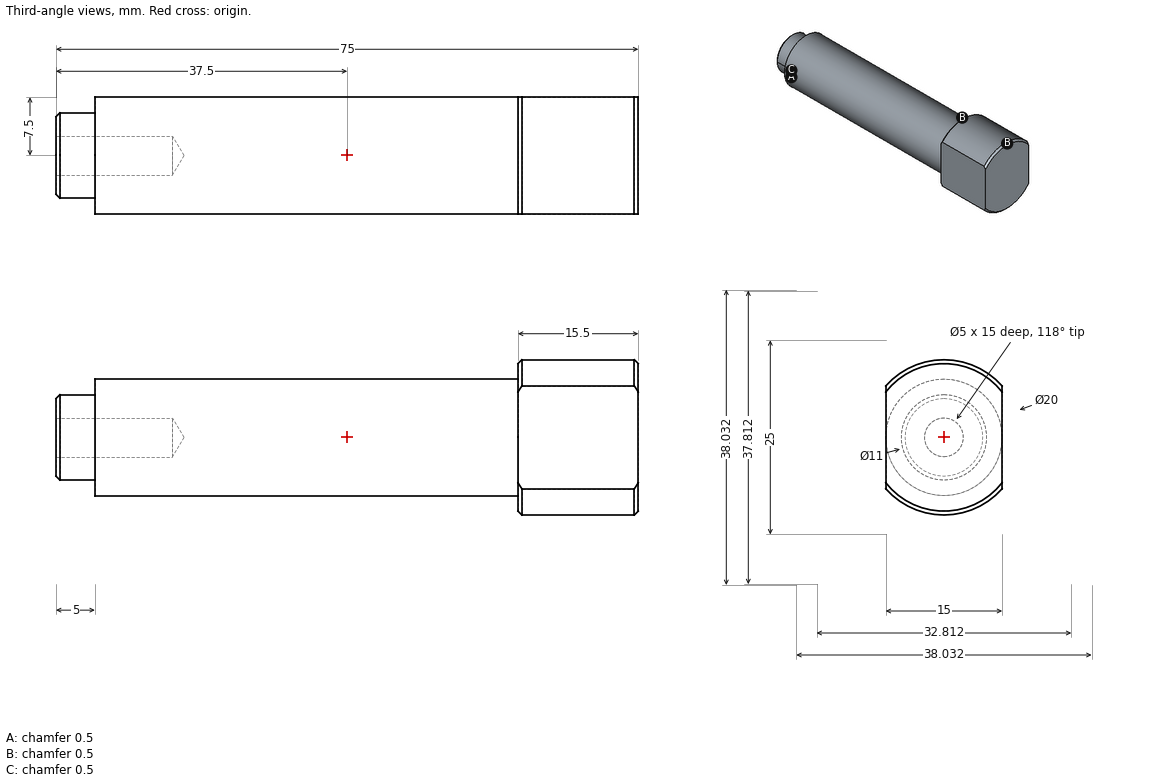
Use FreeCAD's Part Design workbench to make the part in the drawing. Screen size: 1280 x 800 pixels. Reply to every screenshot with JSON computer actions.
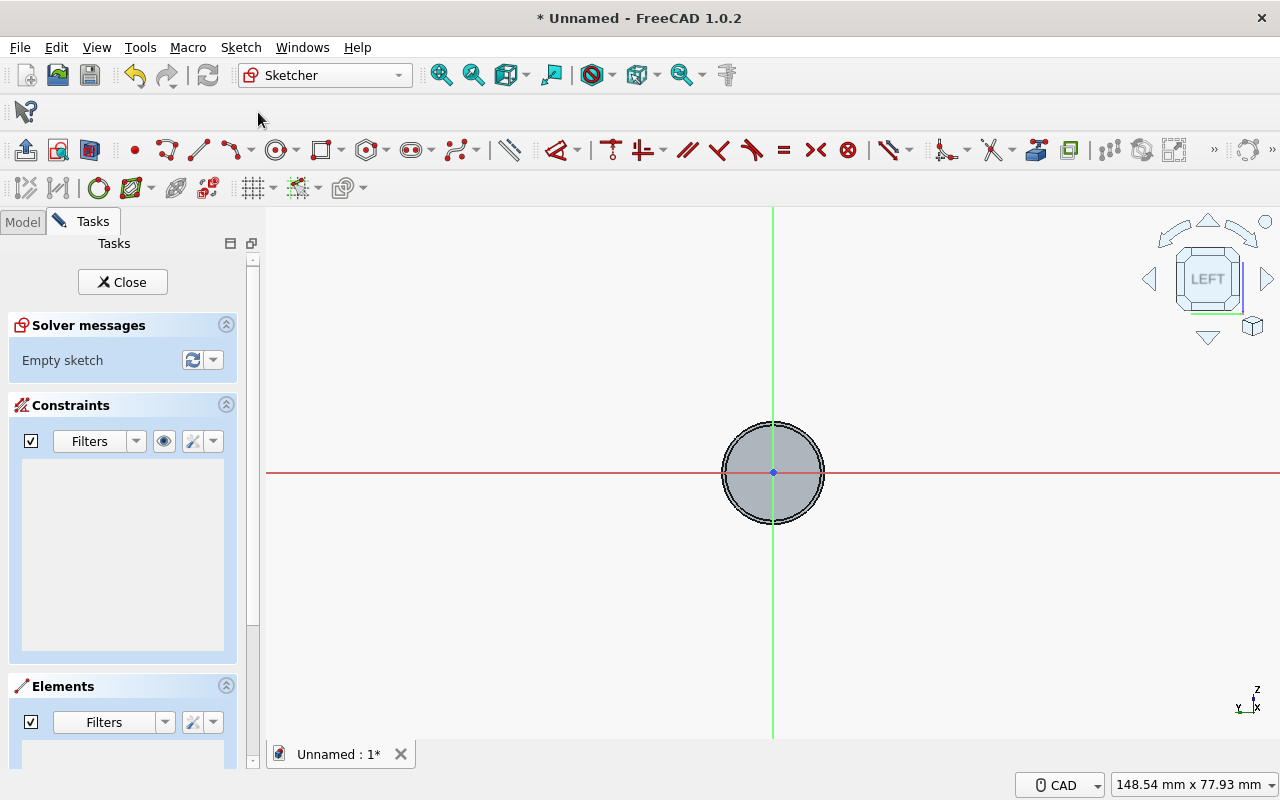
{"action": "scroll", "coordinate": [782, 473], "scroll_direction": "up", "scroll_amount": 11}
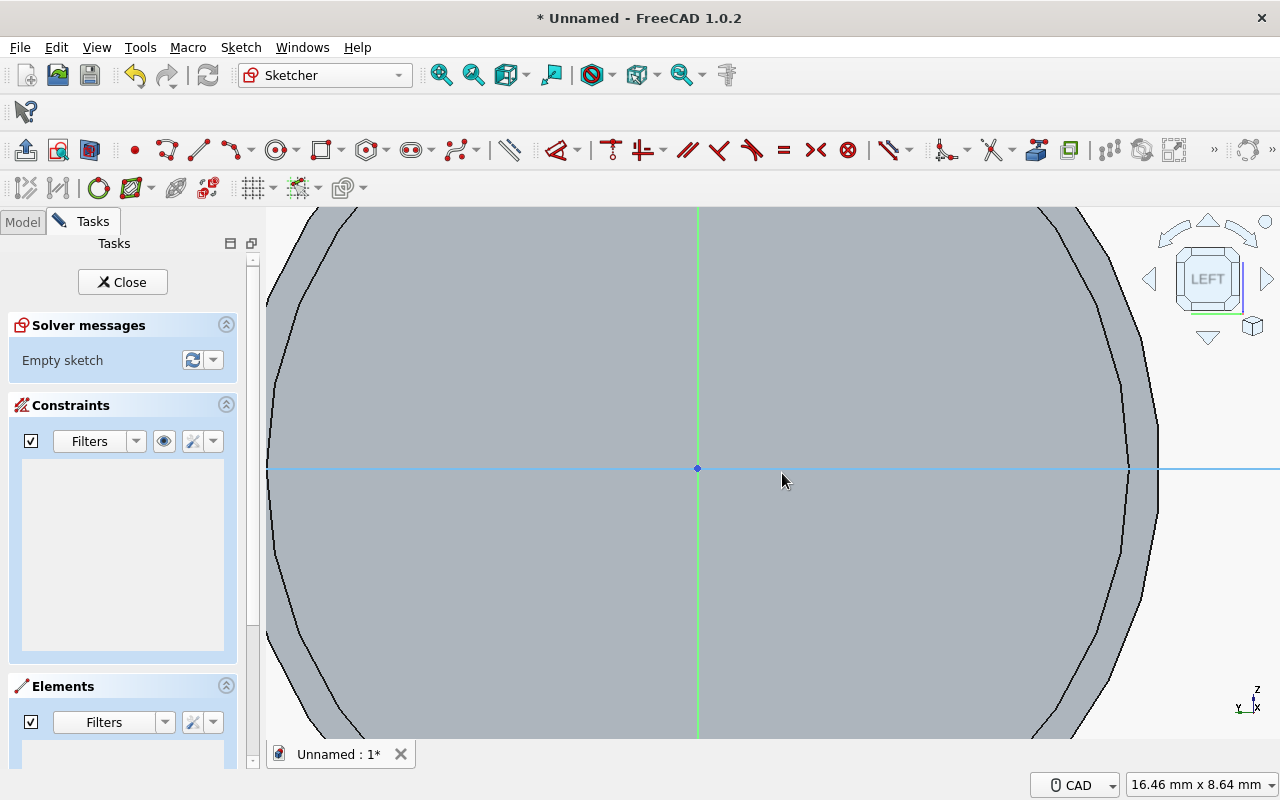
{"action": "left_click", "coordinate": [276, 150]}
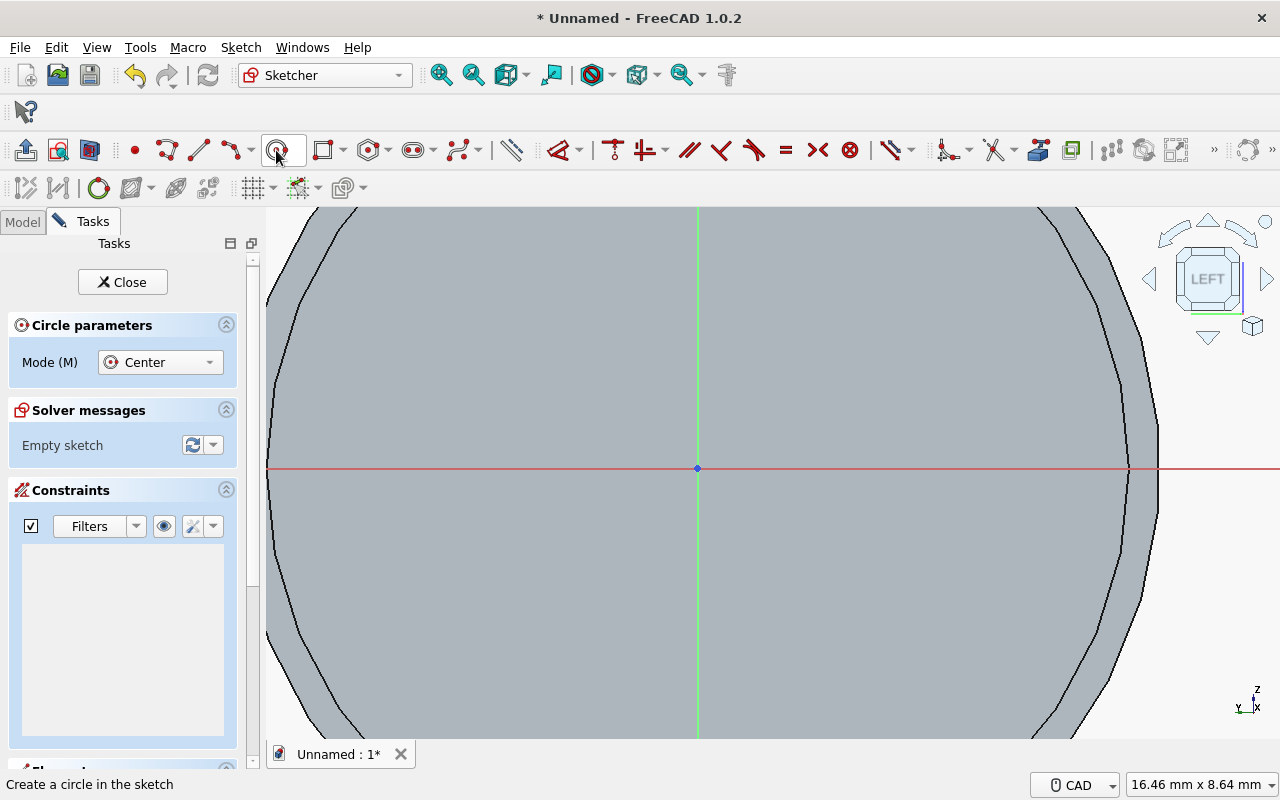
{"action": "left_click", "coordinate": [698, 469]}
{"action": "left_click", "coordinate": [807, 360]}
{"action": "key", "text": "Escape"}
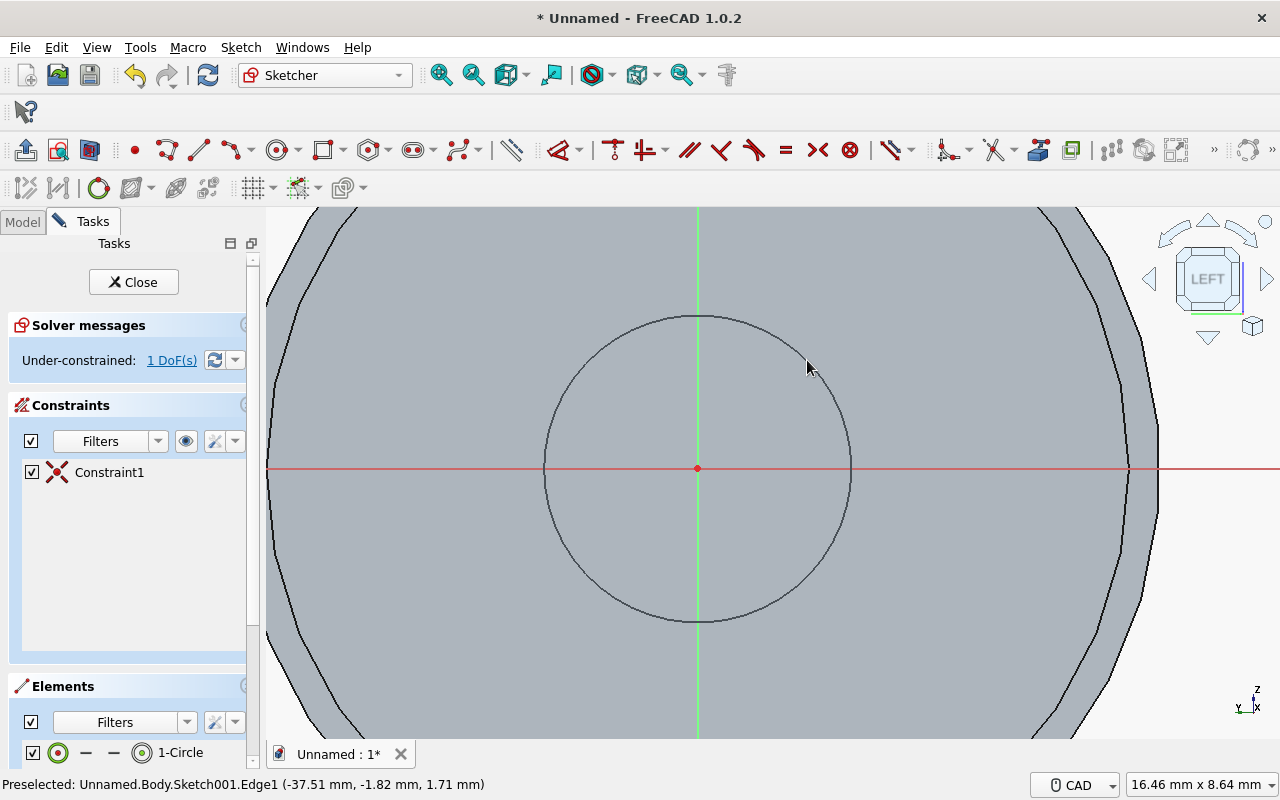
{"action": "left_click", "coordinate": [558, 150]}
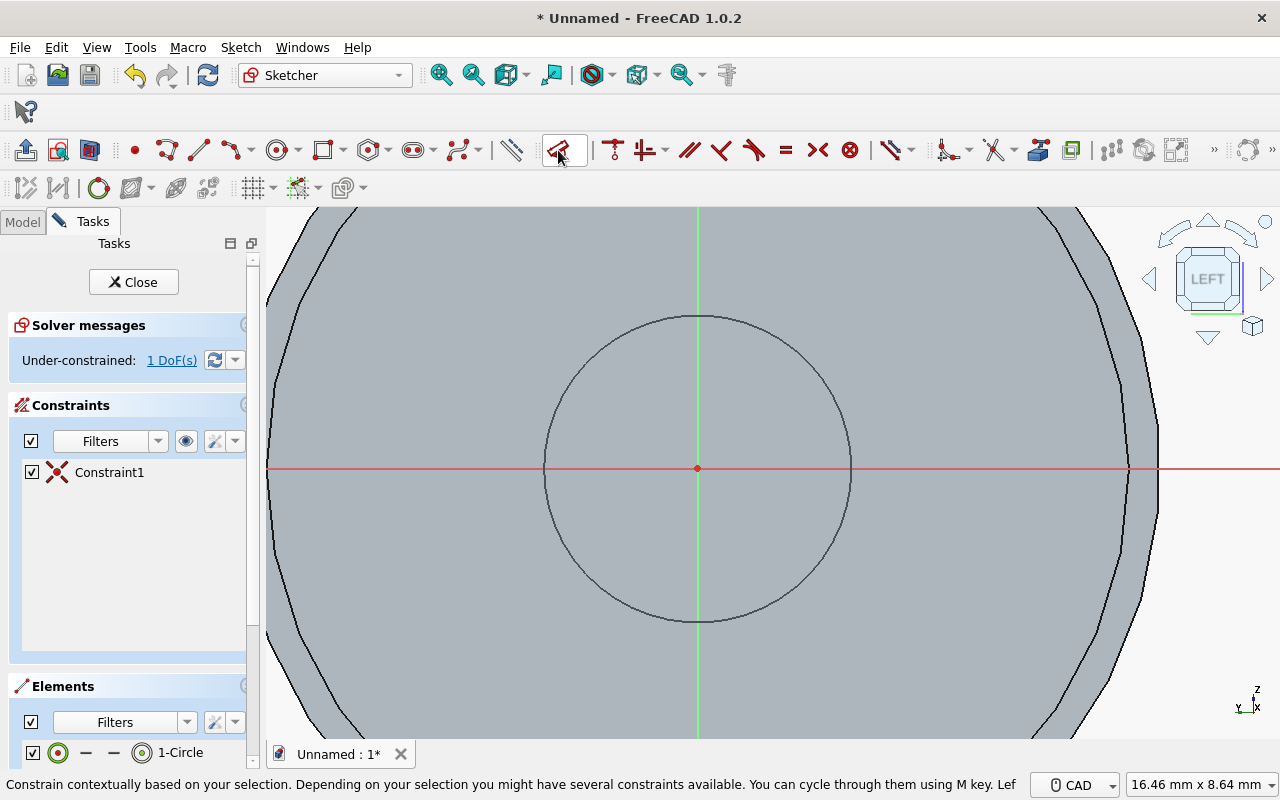
{"action": "left_click", "coordinate": [806, 360]}
{"action": "left_click", "coordinate": [829, 337]}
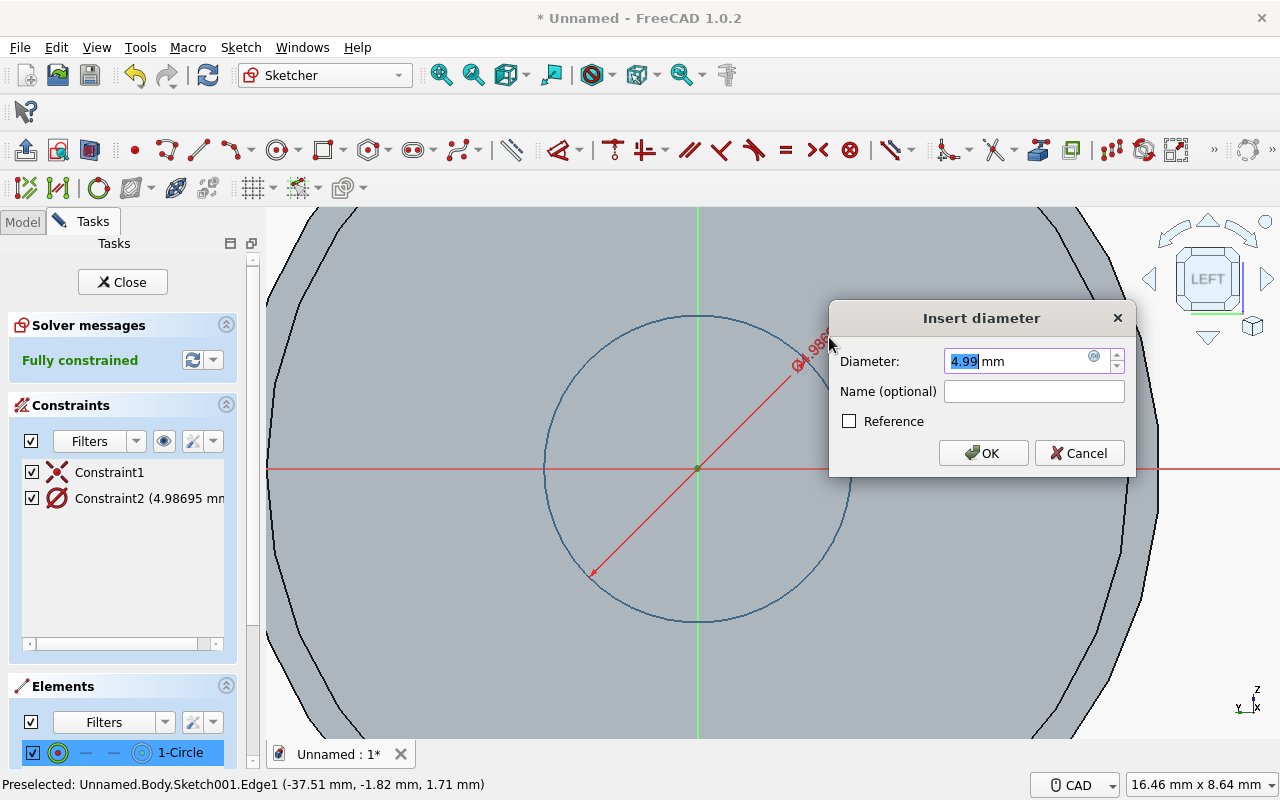
{"action": "type", "text": "5"}
{"action": "key", "text": "Return"}
{"action": "key", "text": "Escape"}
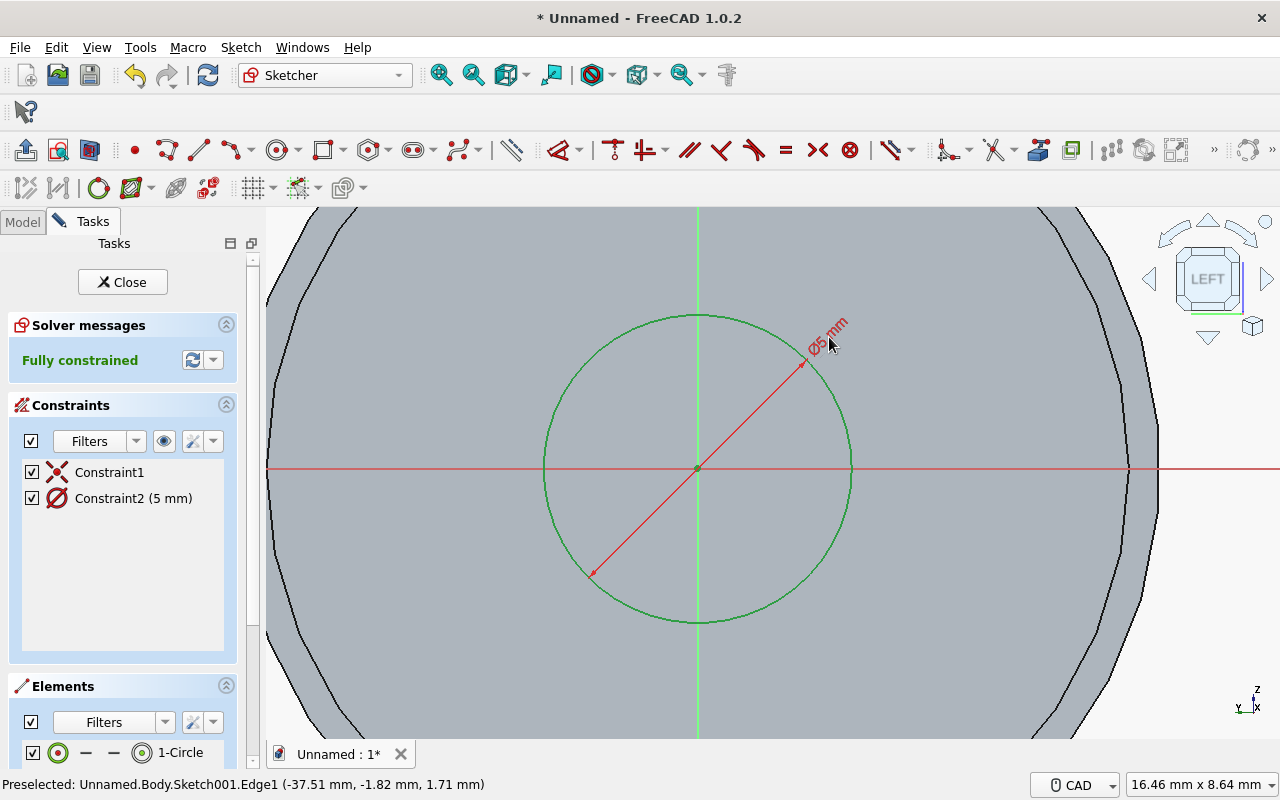
{"action": "left_click", "coordinate": [123, 282]}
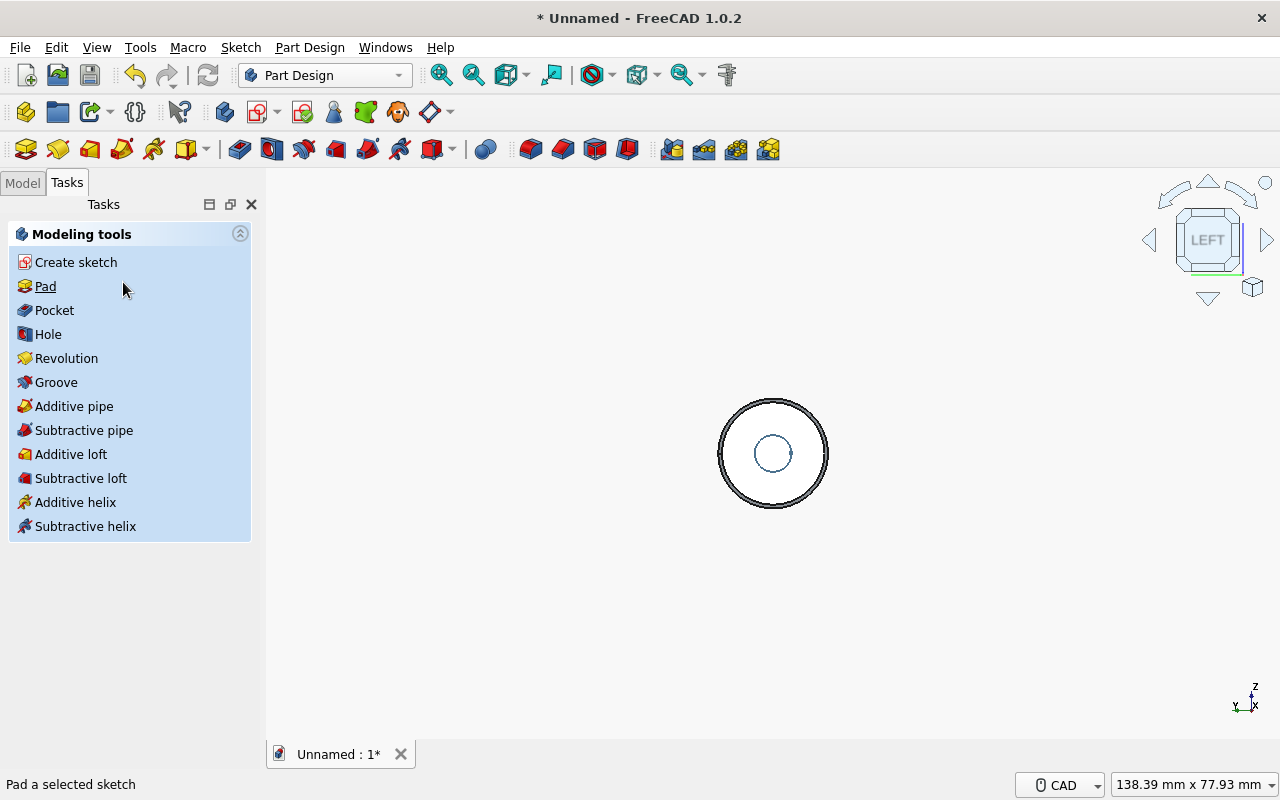
{"action": "left_click", "coordinate": [272, 150]}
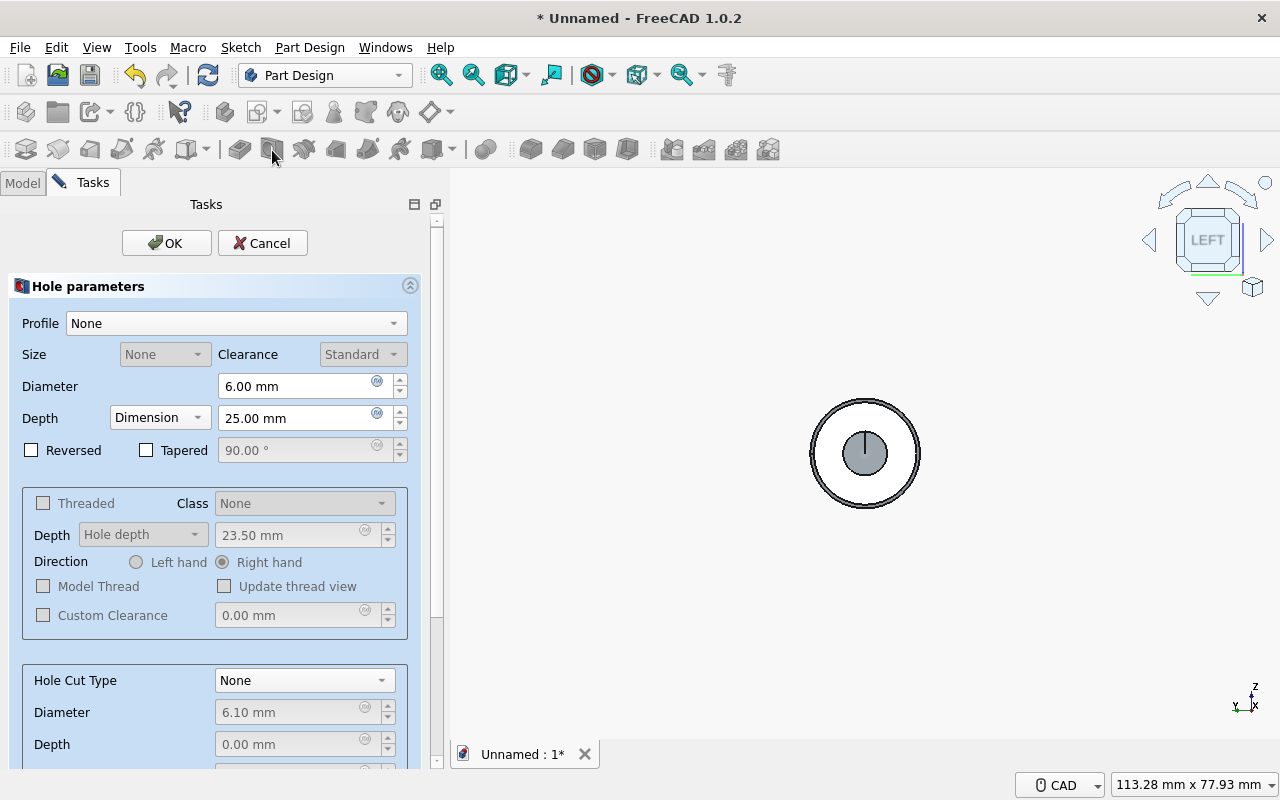
{"action": "triple_click", "coordinate": [305, 386]}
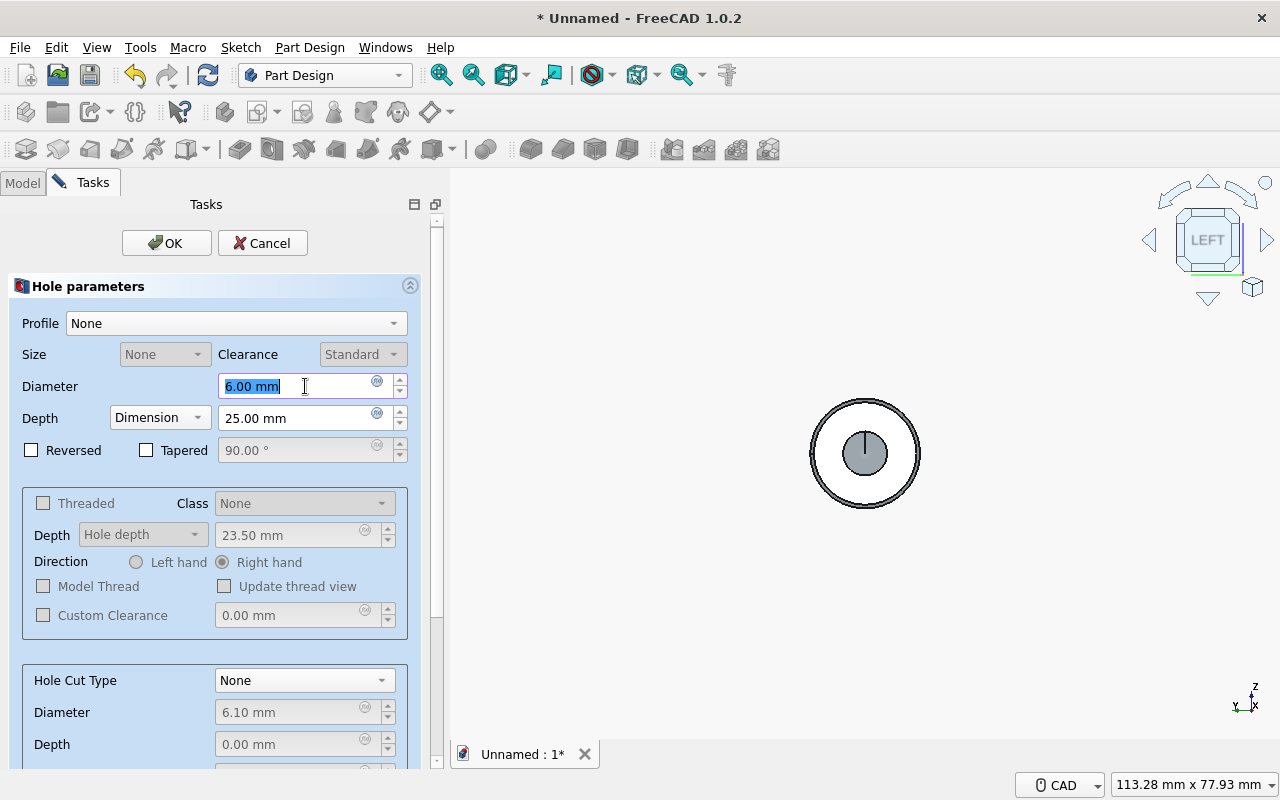
{"action": "type", "text": "5"}
{"action": "key", "text": "Tab"}